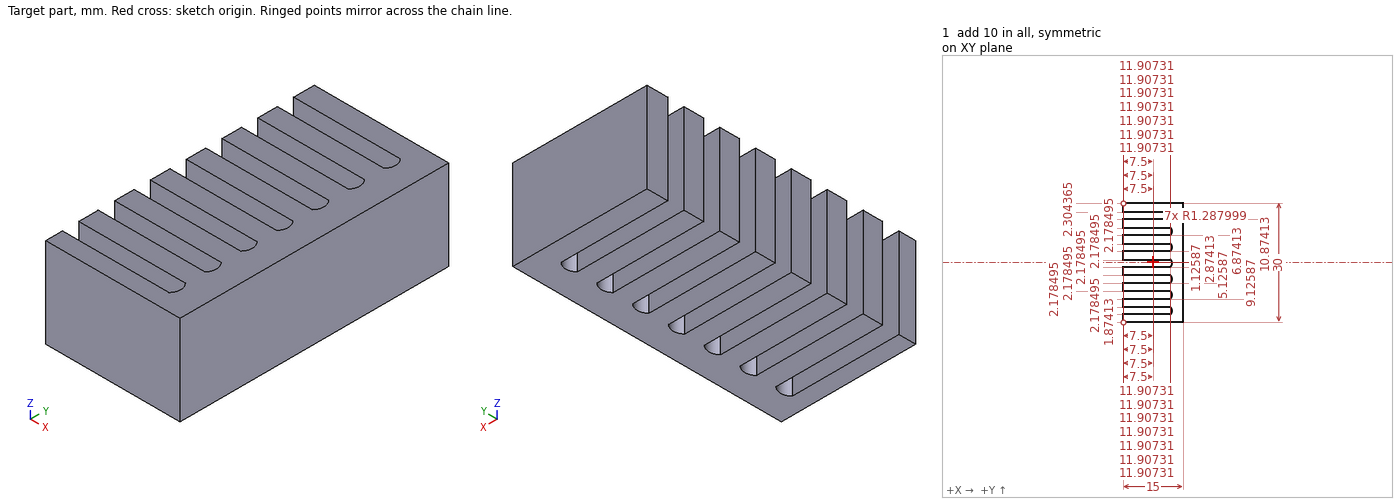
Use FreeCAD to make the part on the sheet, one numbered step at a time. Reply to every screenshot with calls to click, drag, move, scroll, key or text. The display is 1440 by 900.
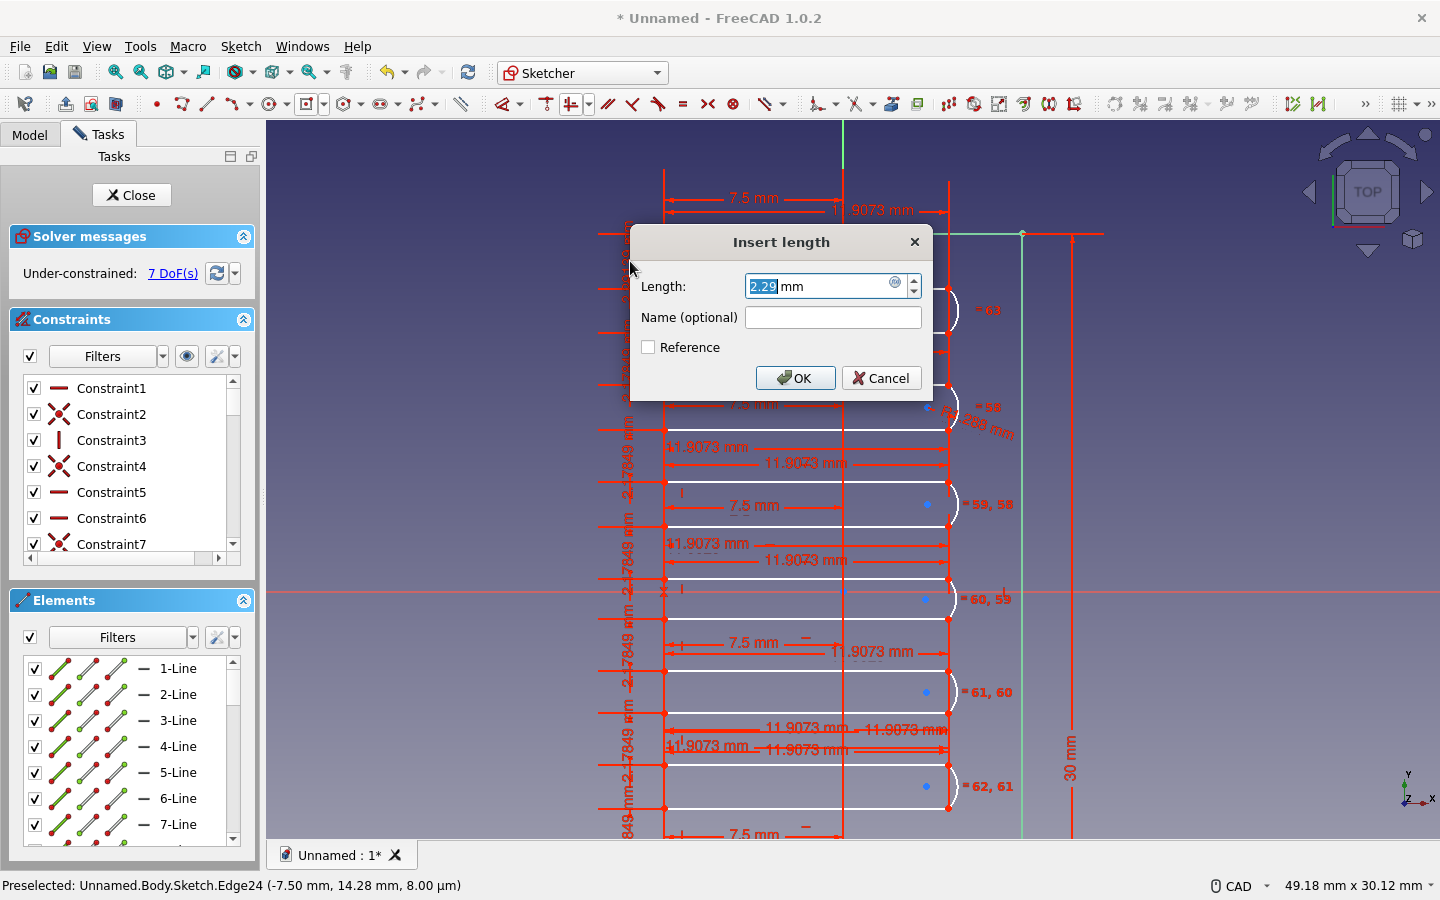
text(2.304365)
key(Return)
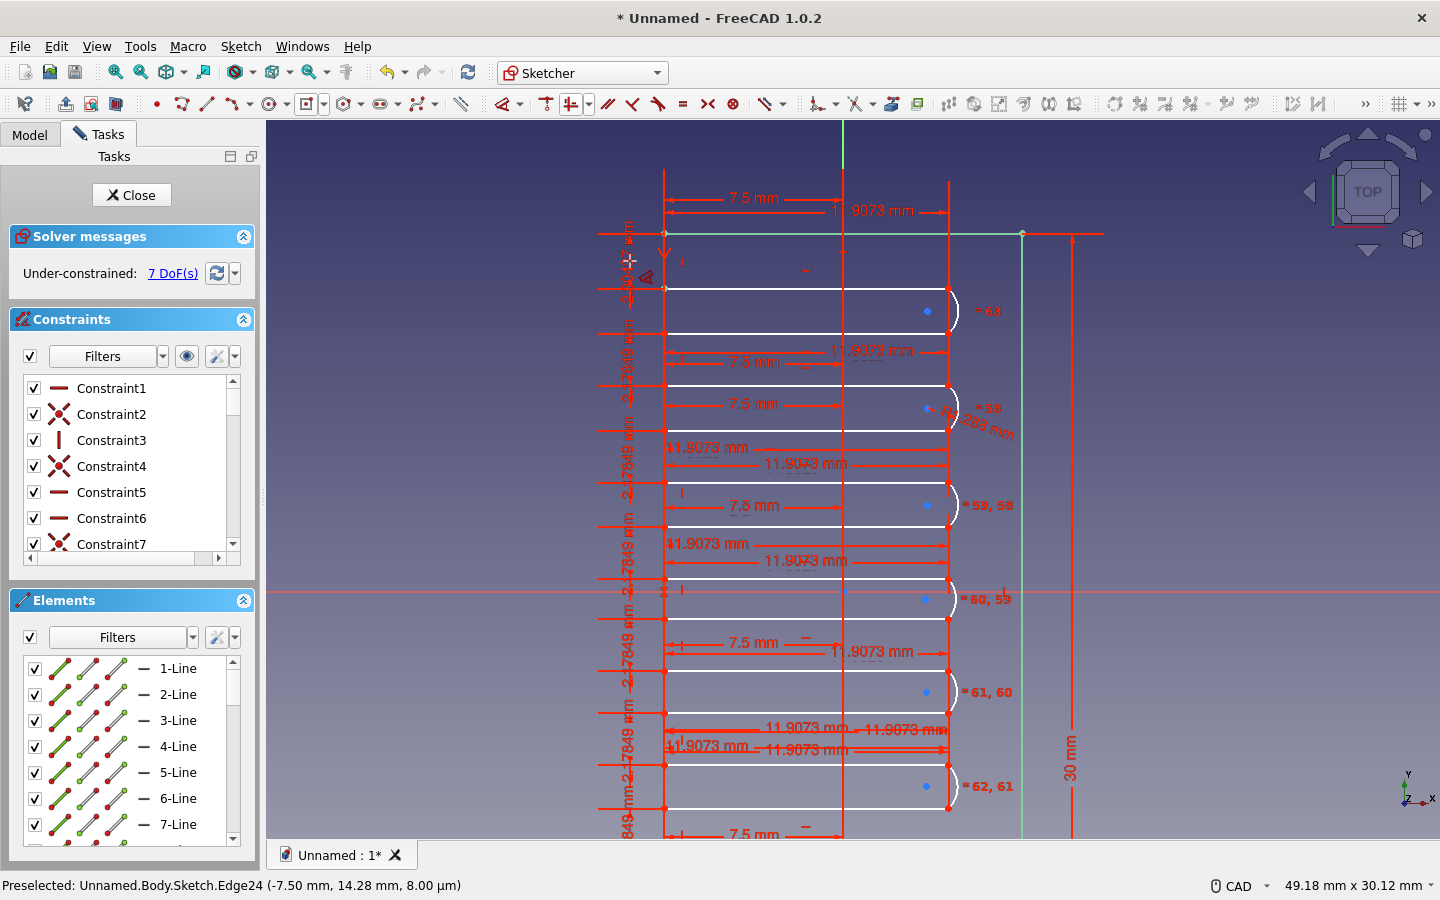
click(750, 289)
click(806, 255)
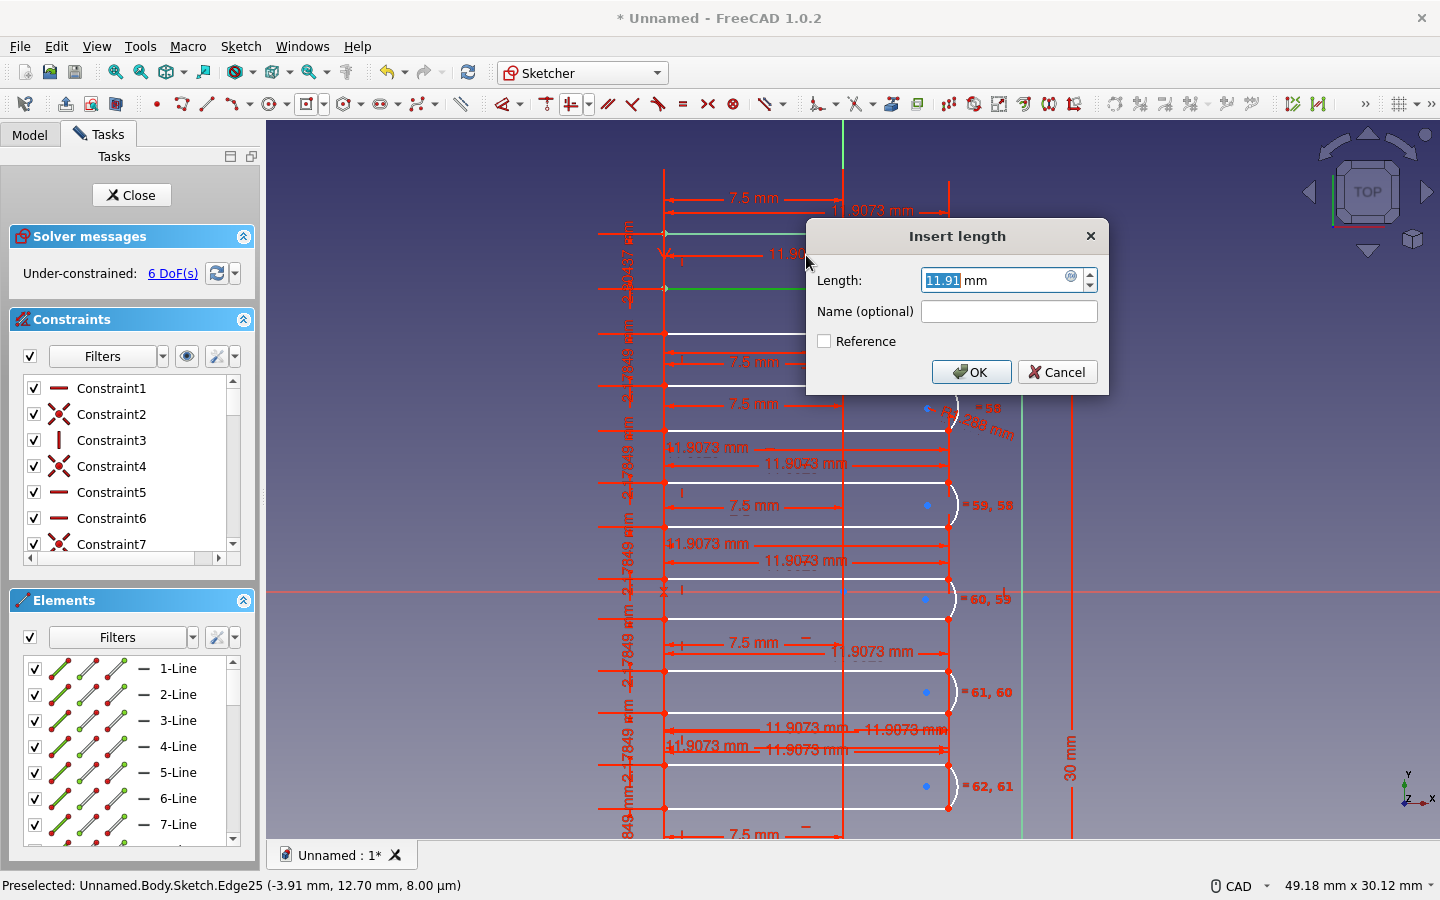
text(11.90731)
key(Return)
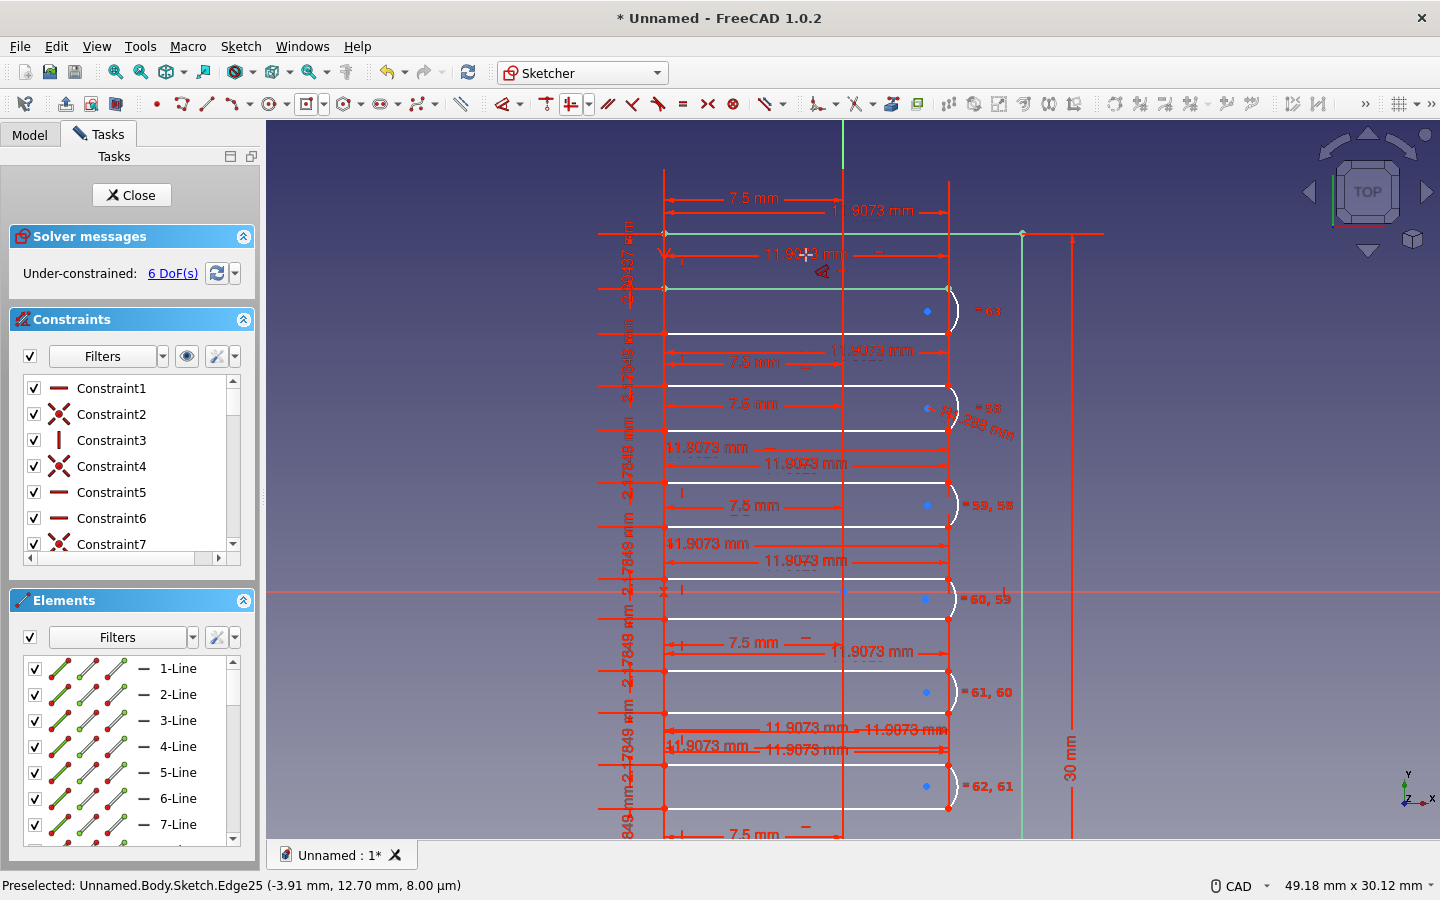
click(949, 431)
click(983, 511)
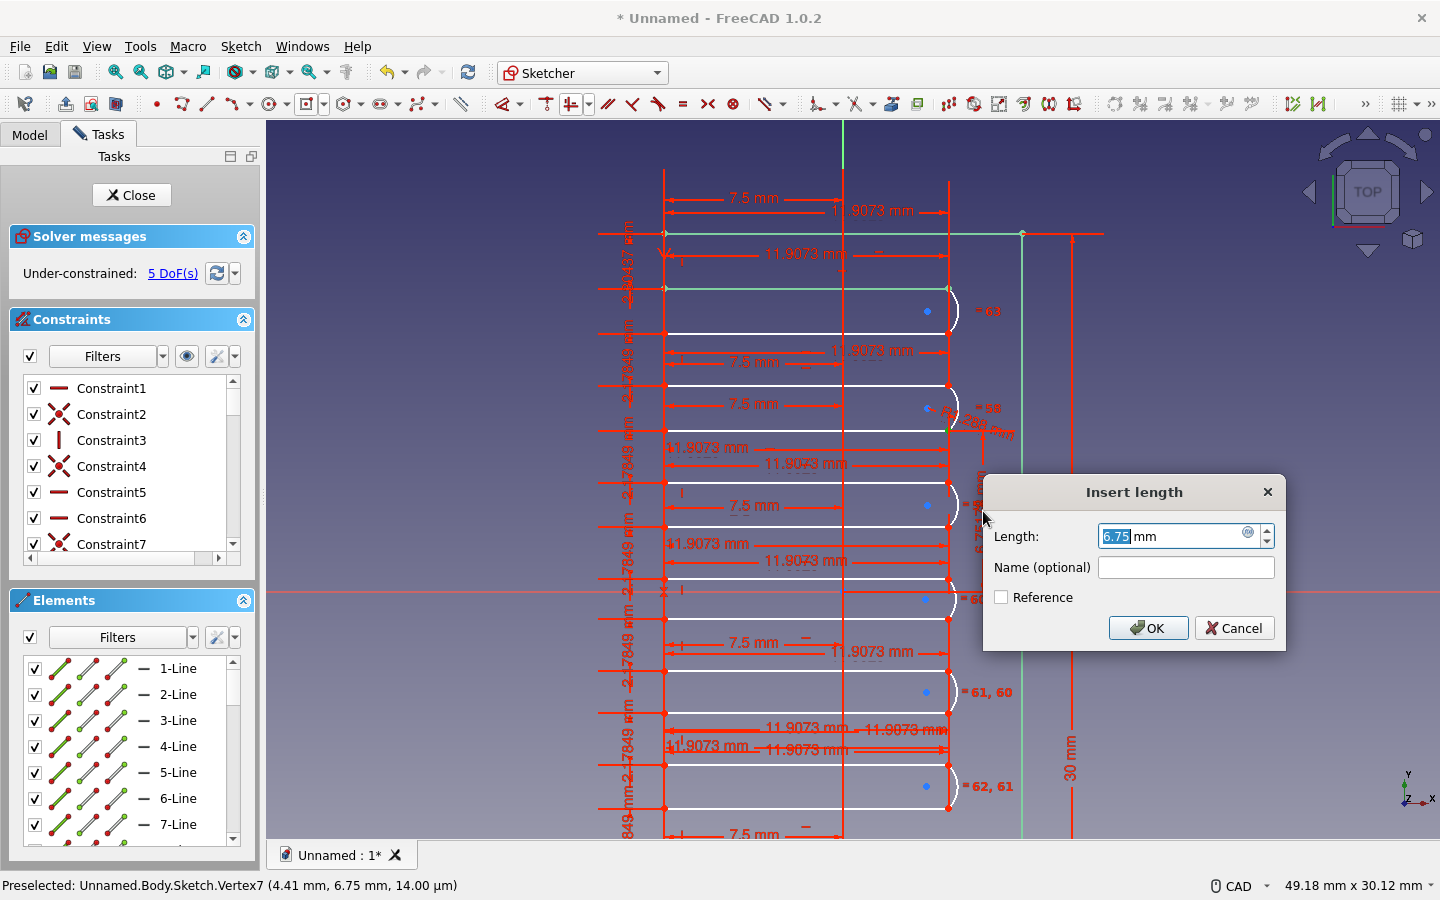
text(6.87413)
key(Return)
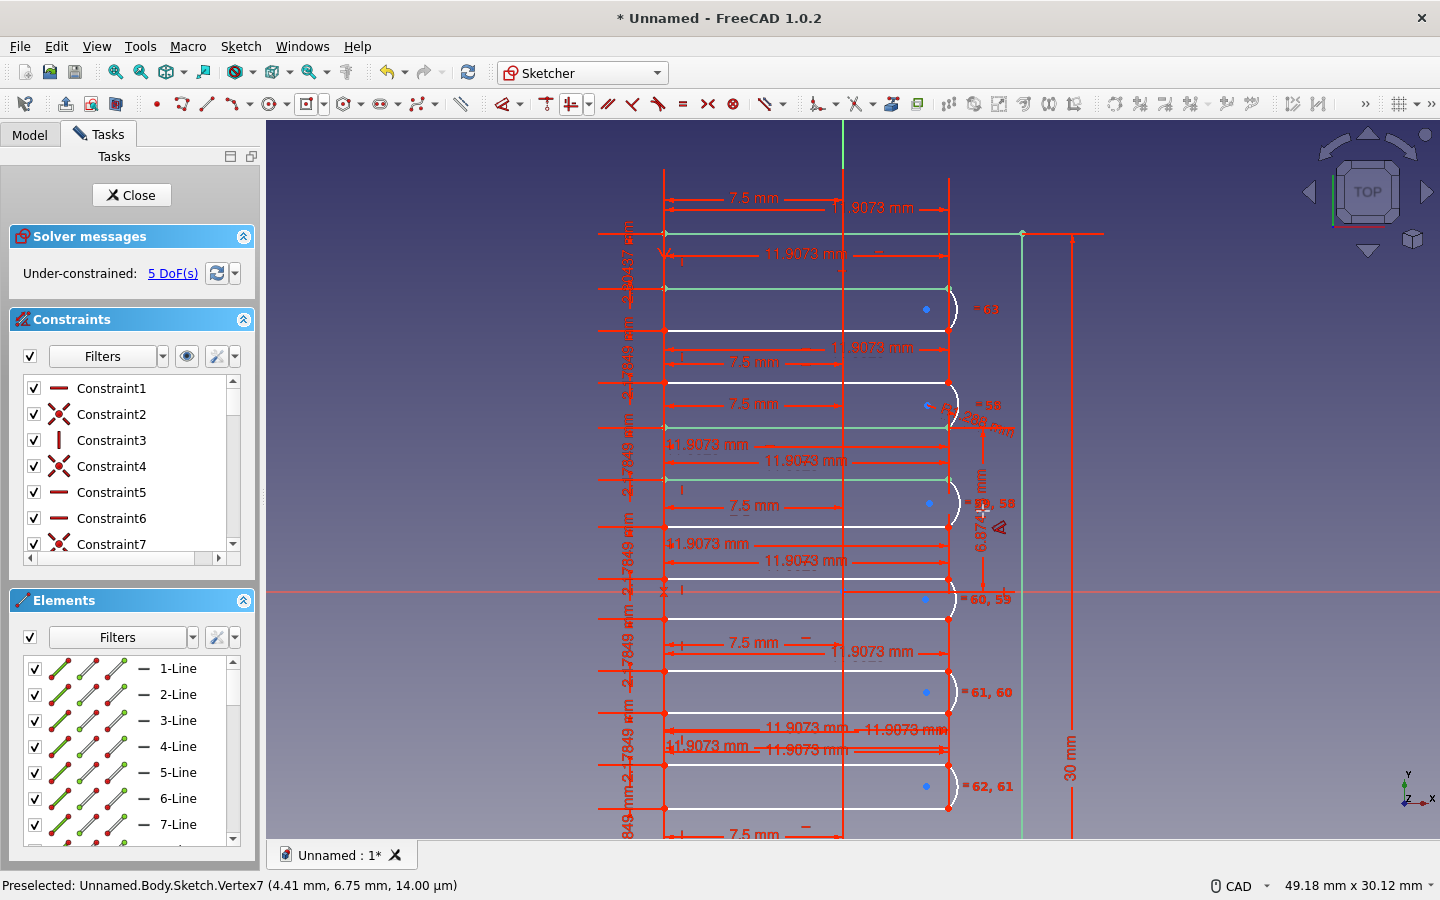
click(949, 527)
click(983, 560)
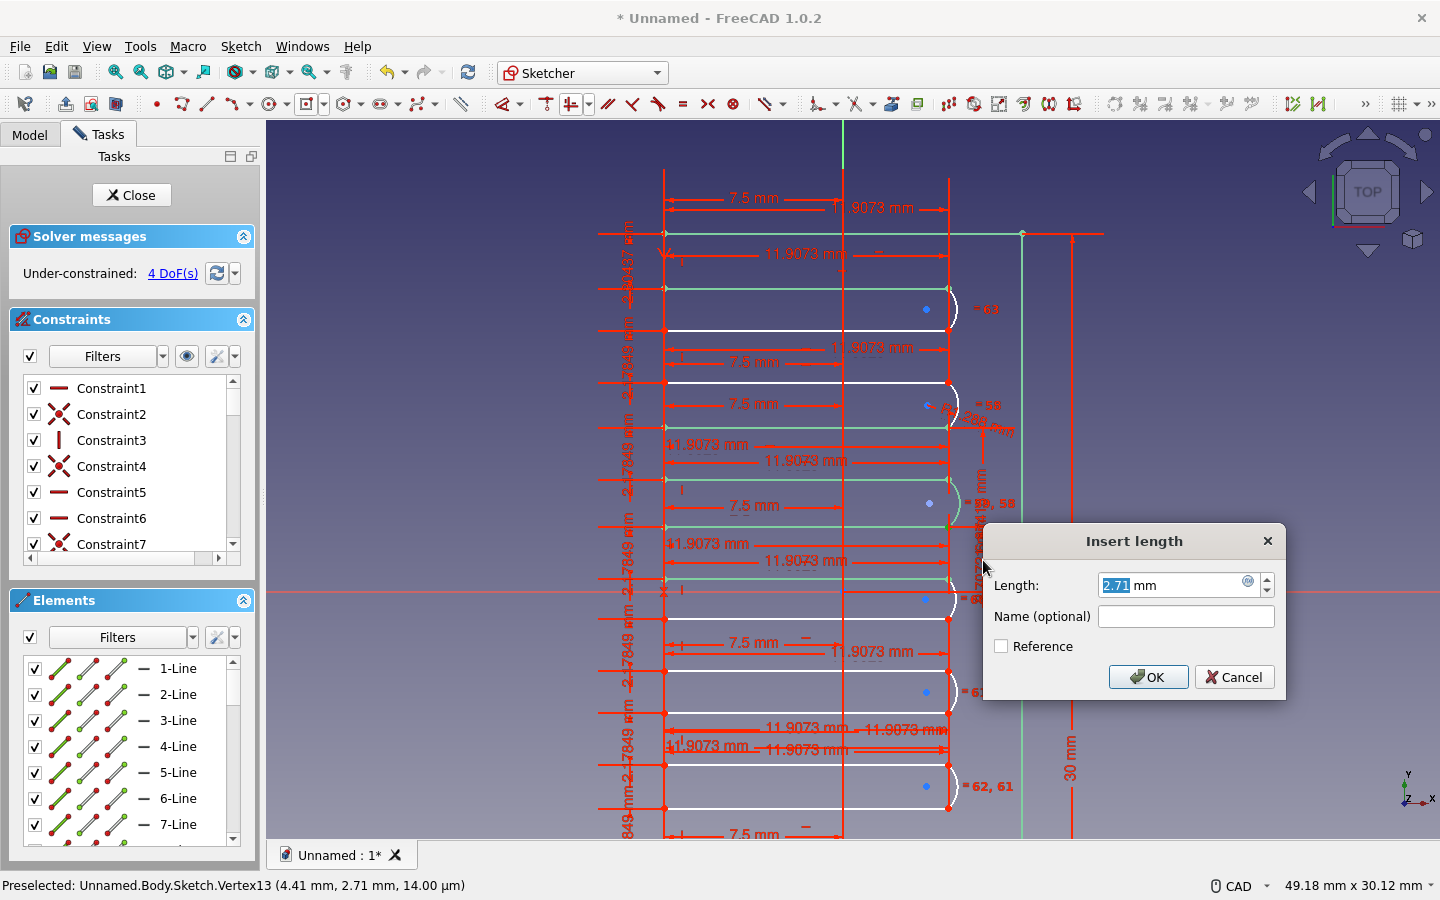
text(2.87413)
key(Return)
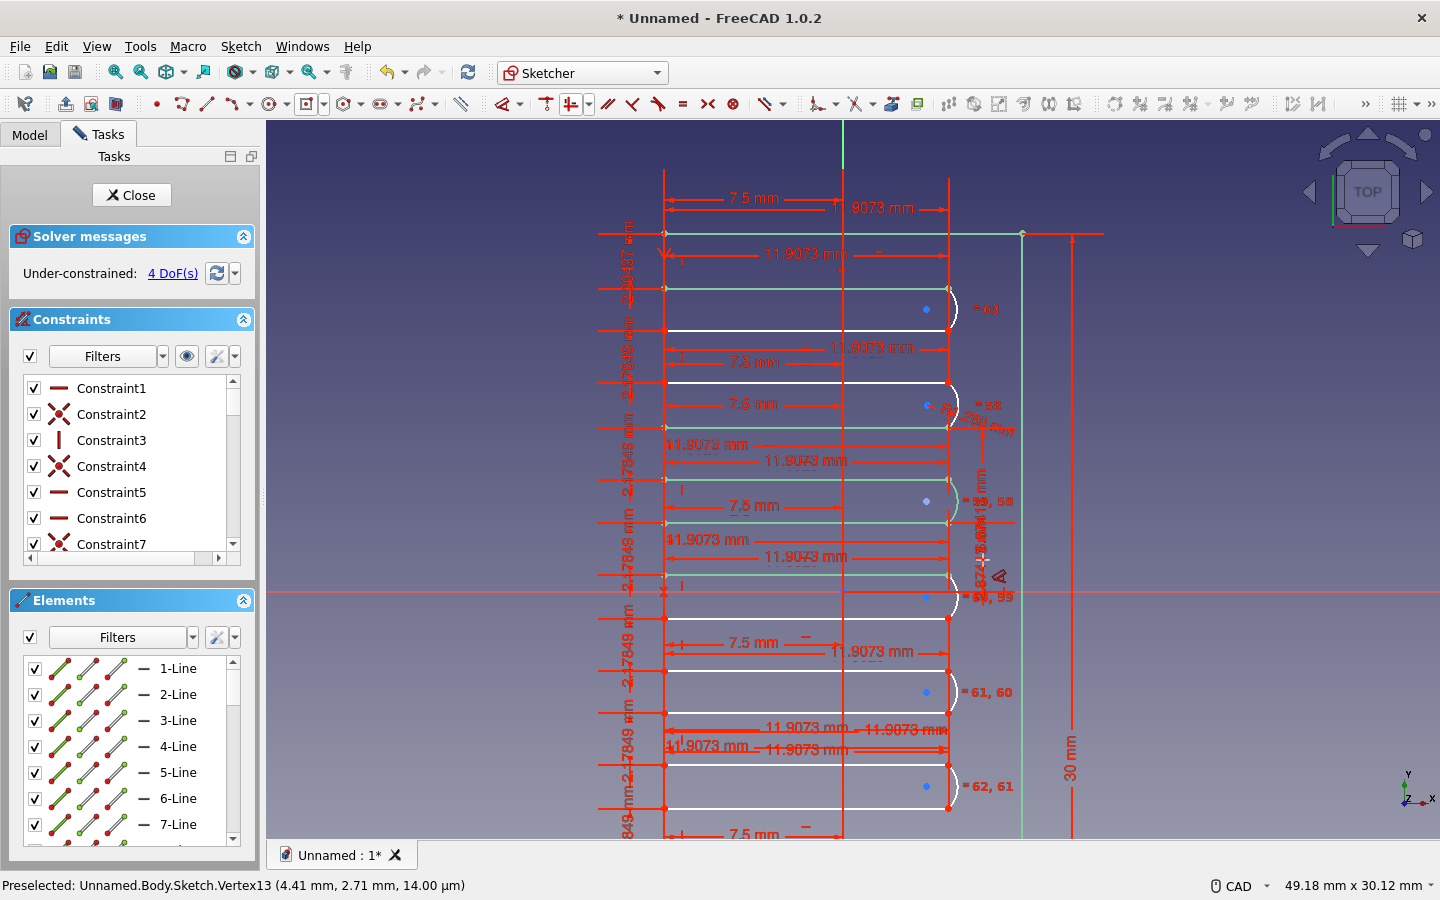
scroll(949, 619, up, 2)